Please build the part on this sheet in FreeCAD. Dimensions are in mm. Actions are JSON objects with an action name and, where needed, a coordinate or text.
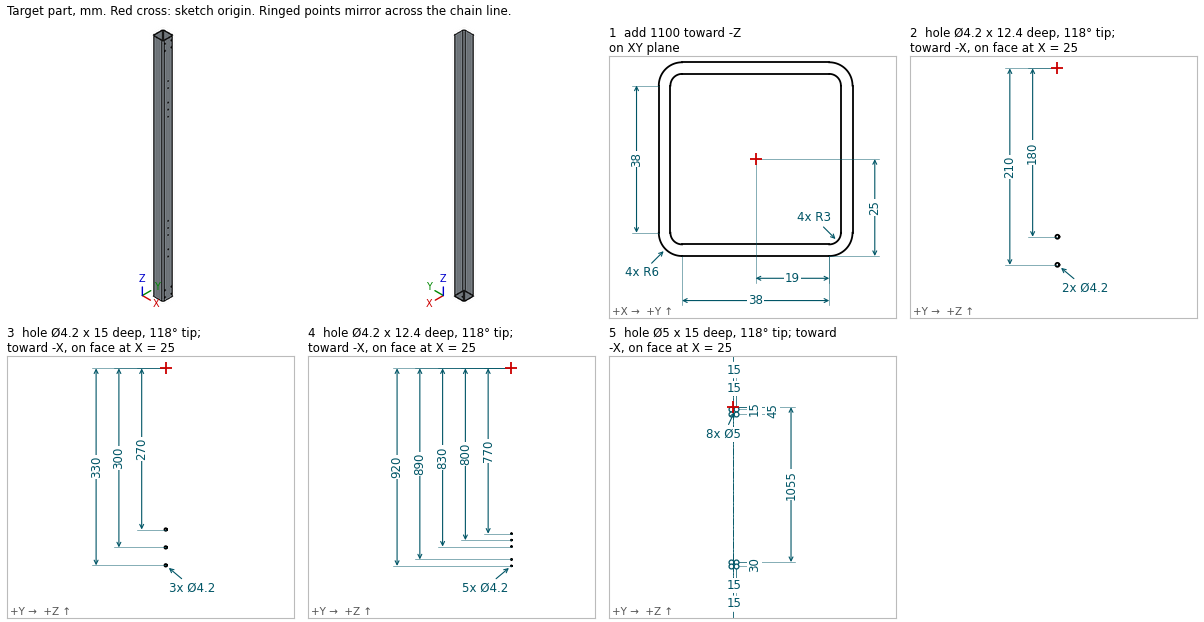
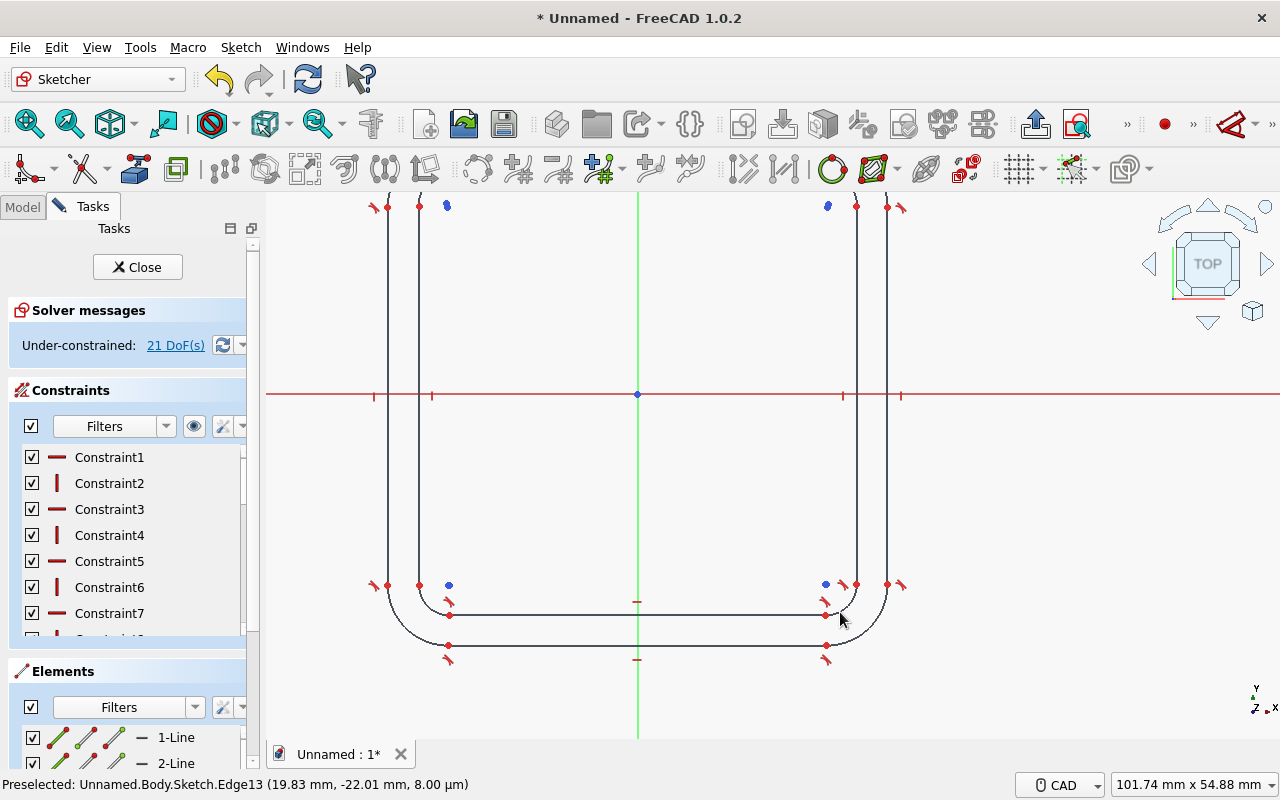
{"action": "left_click", "coordinate": [857, 471]}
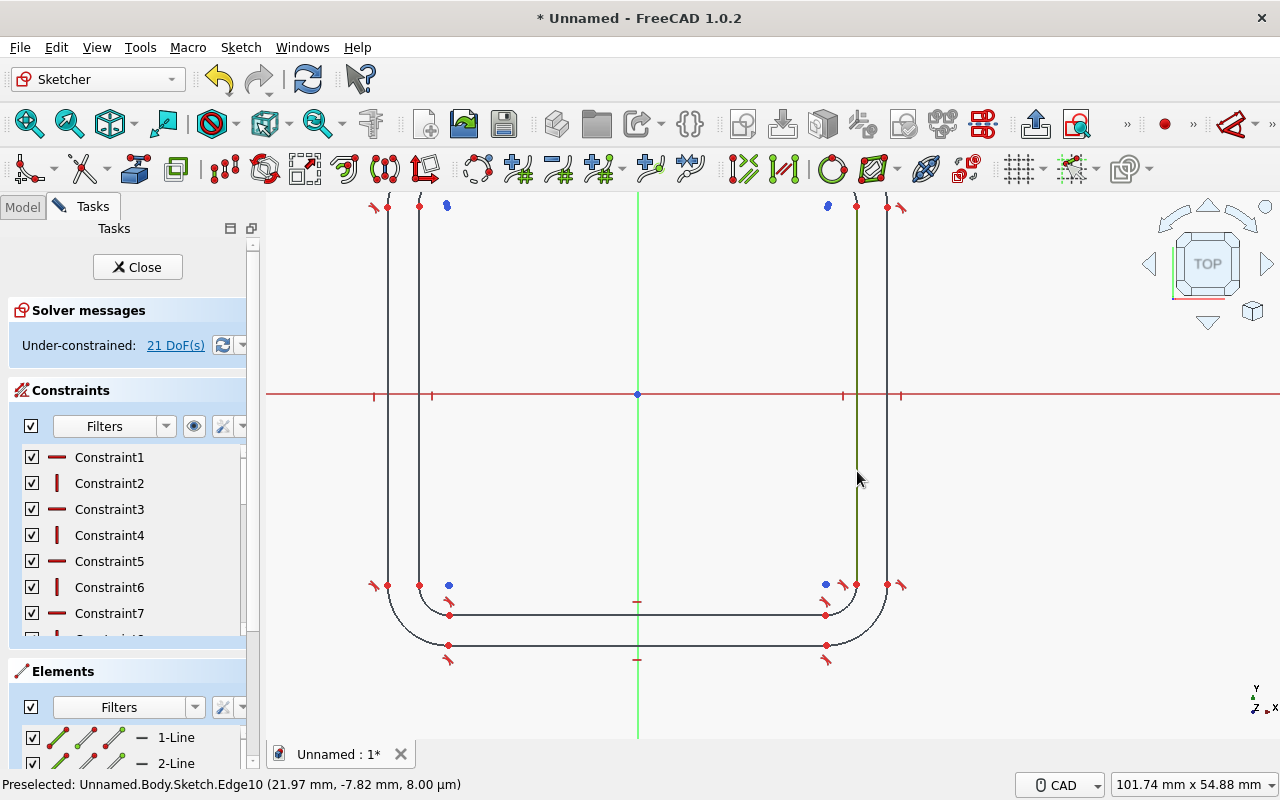
{"action": "scroll", "coordinate": [840, 611], "scroll_direction": "down", "scroll_amount": 2}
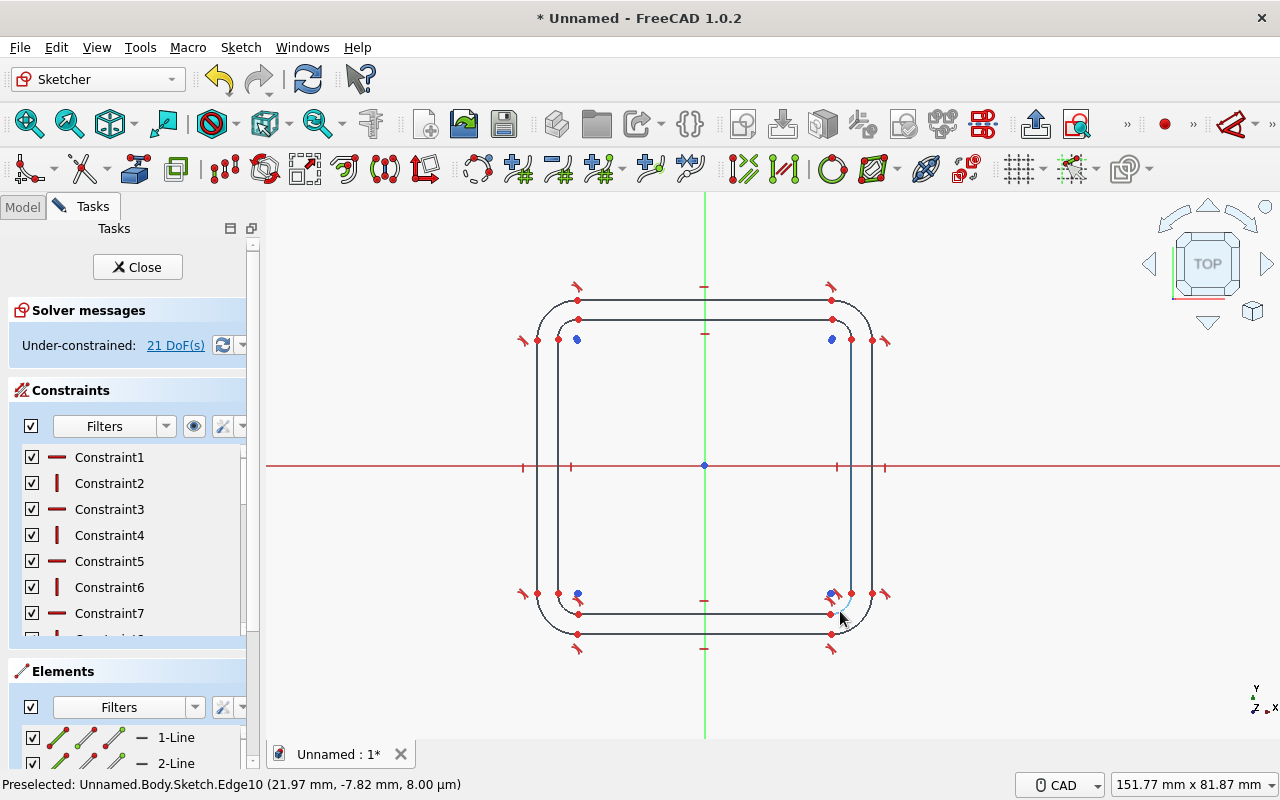
{"action": "scroll", "coordinate": [850, 331], "scroll_direction": "up", "scroll_amount": 2}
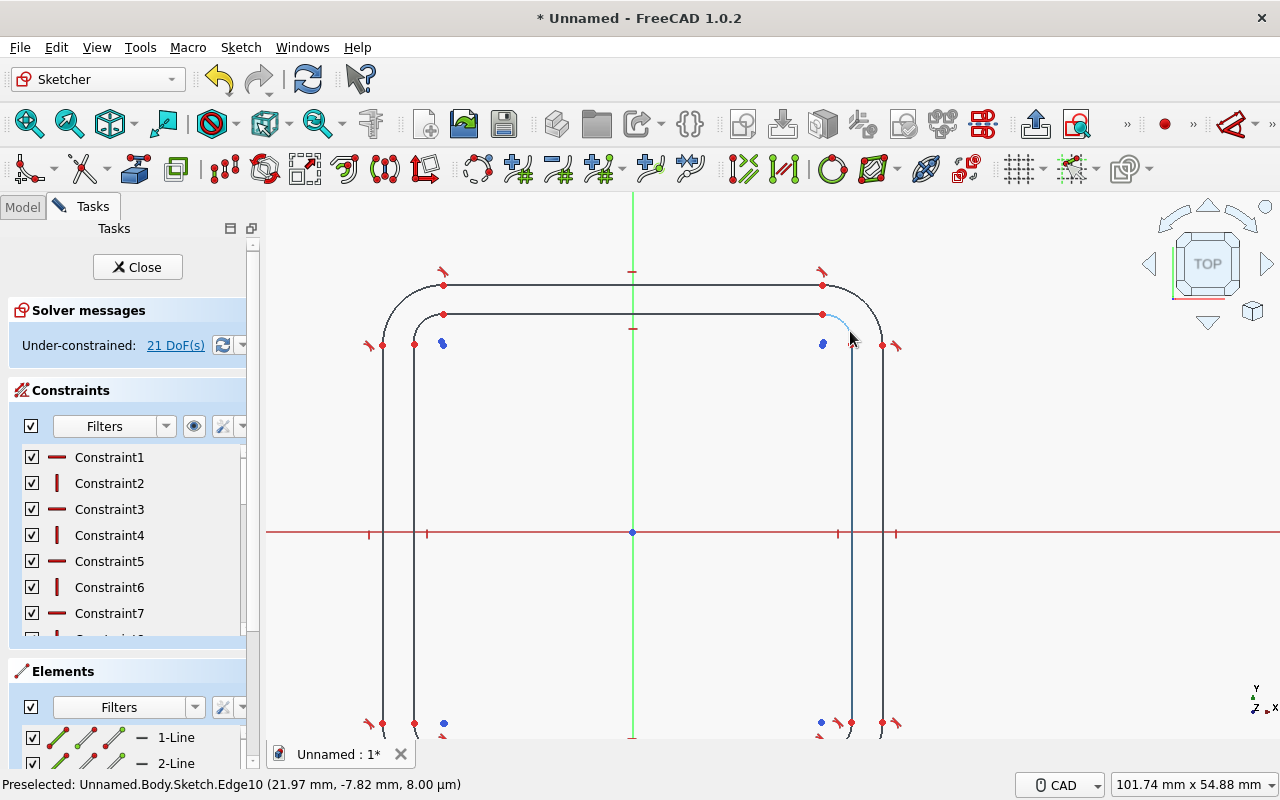
{"action": "left_click", "coordinate": [849, 331]}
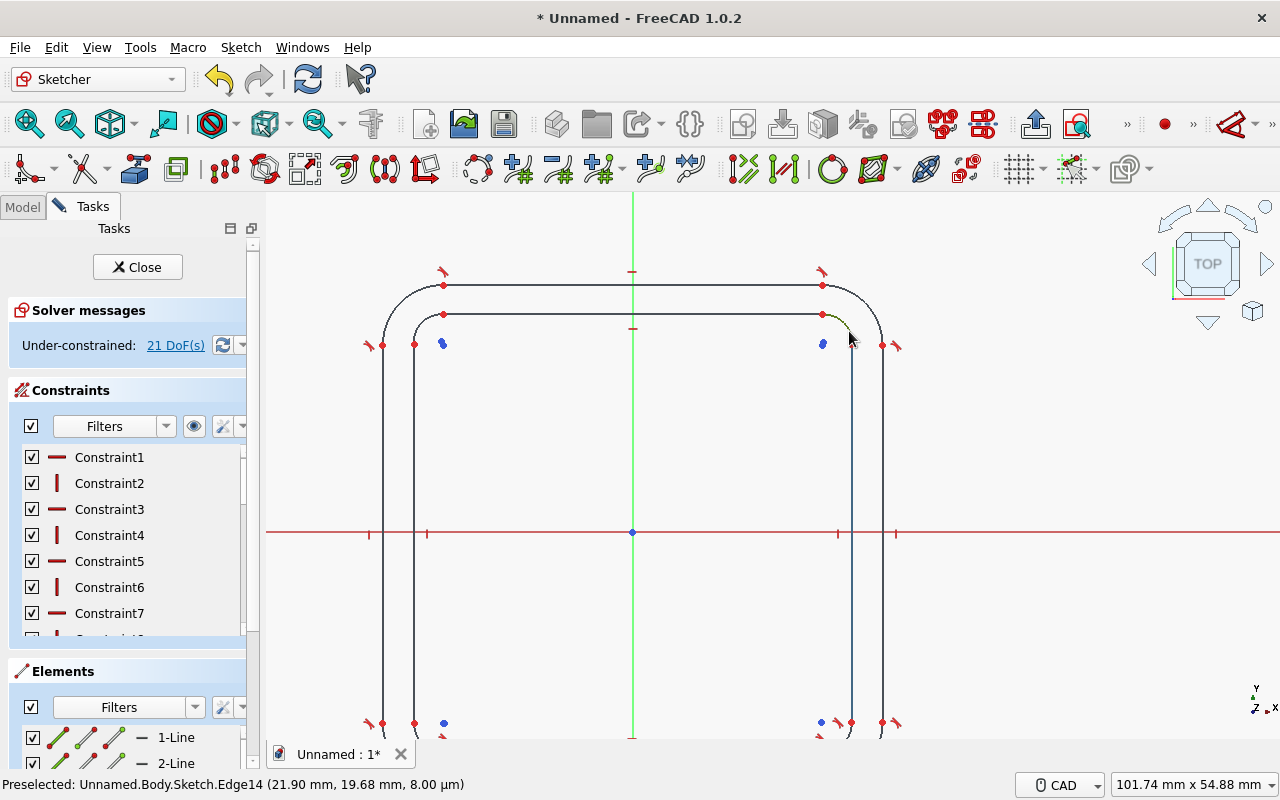
{"action": "key", "text": "t"}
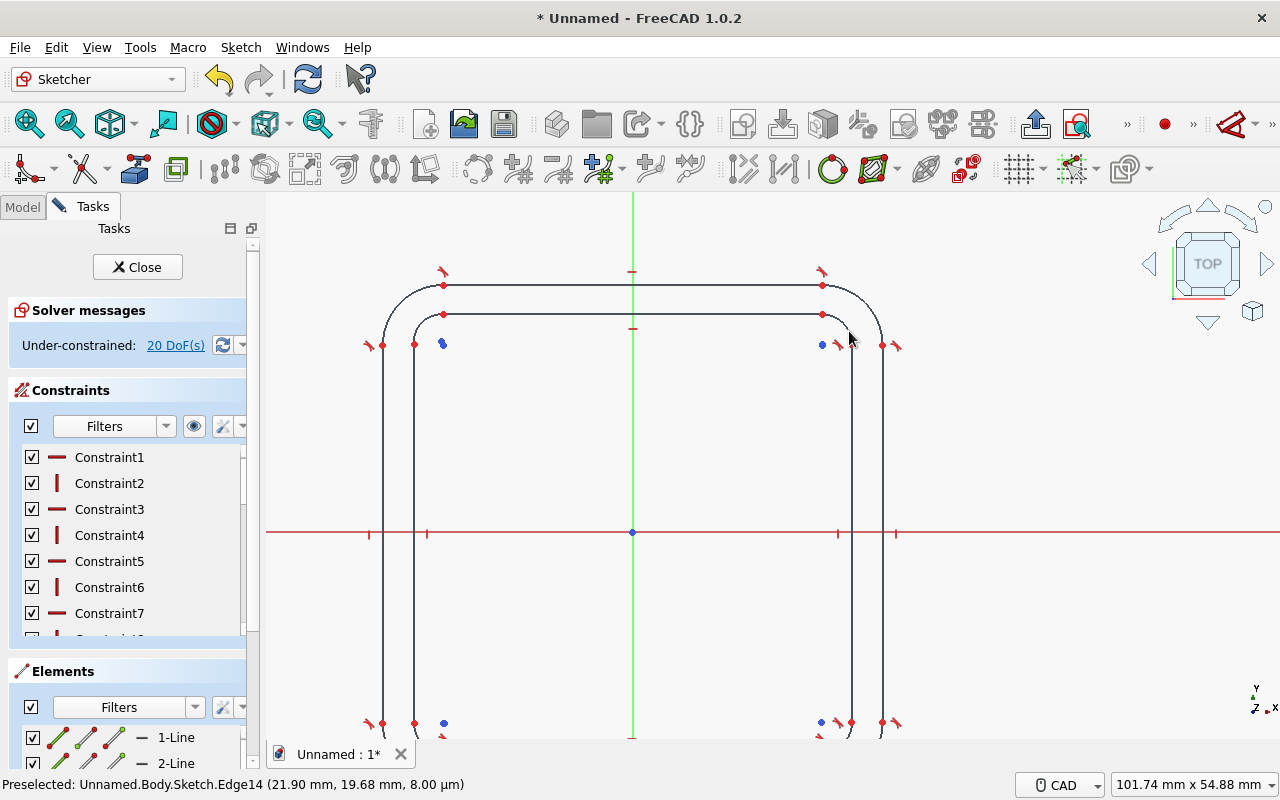
{"action": "left_click", "coordinate": [709, 314]}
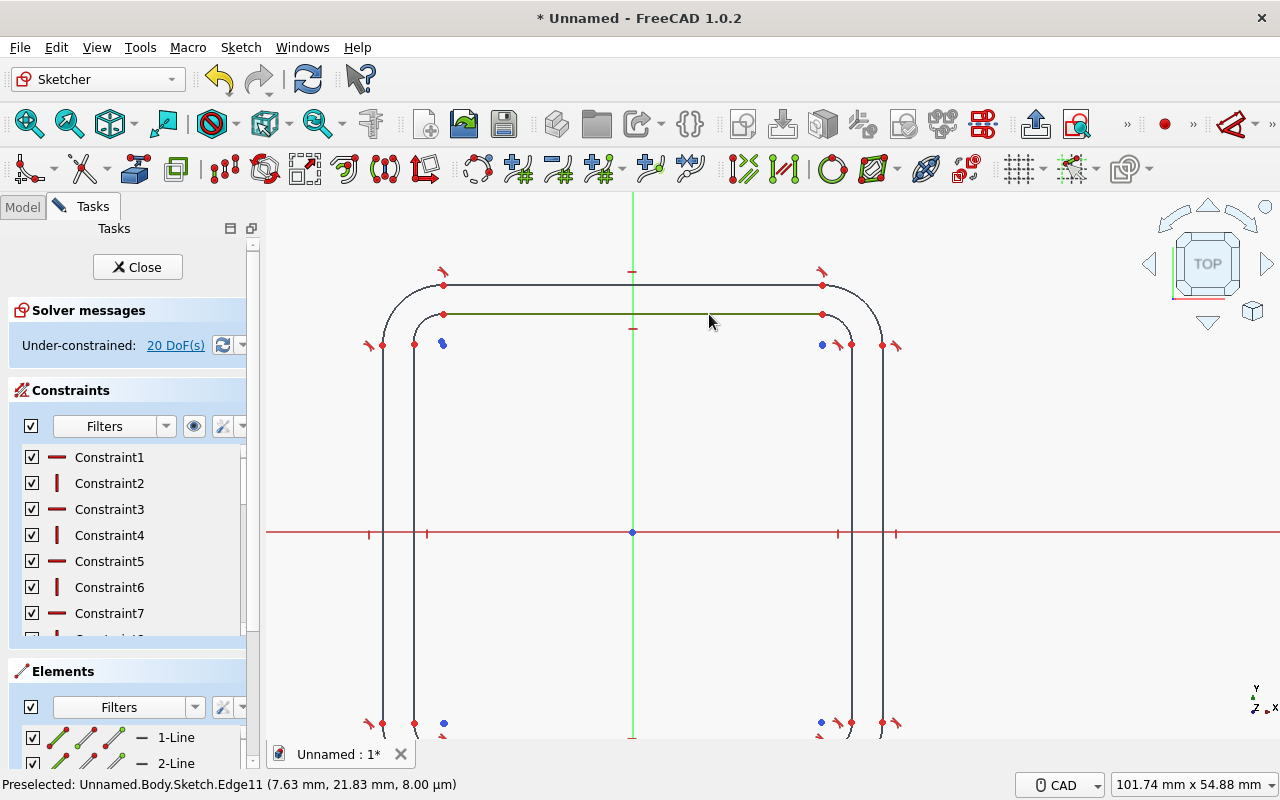
{"action": "left_click", "coordinate": [849, 331]}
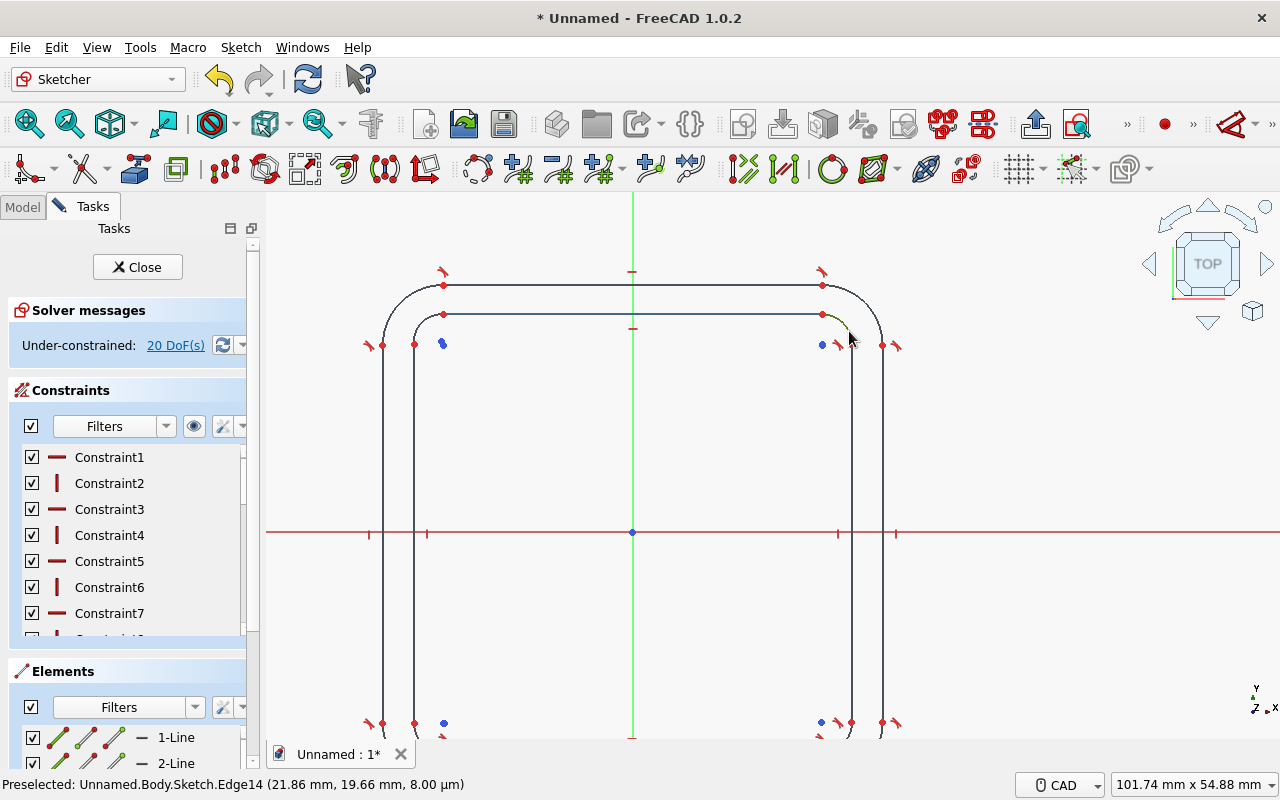
{"action": "key", "text": "t"}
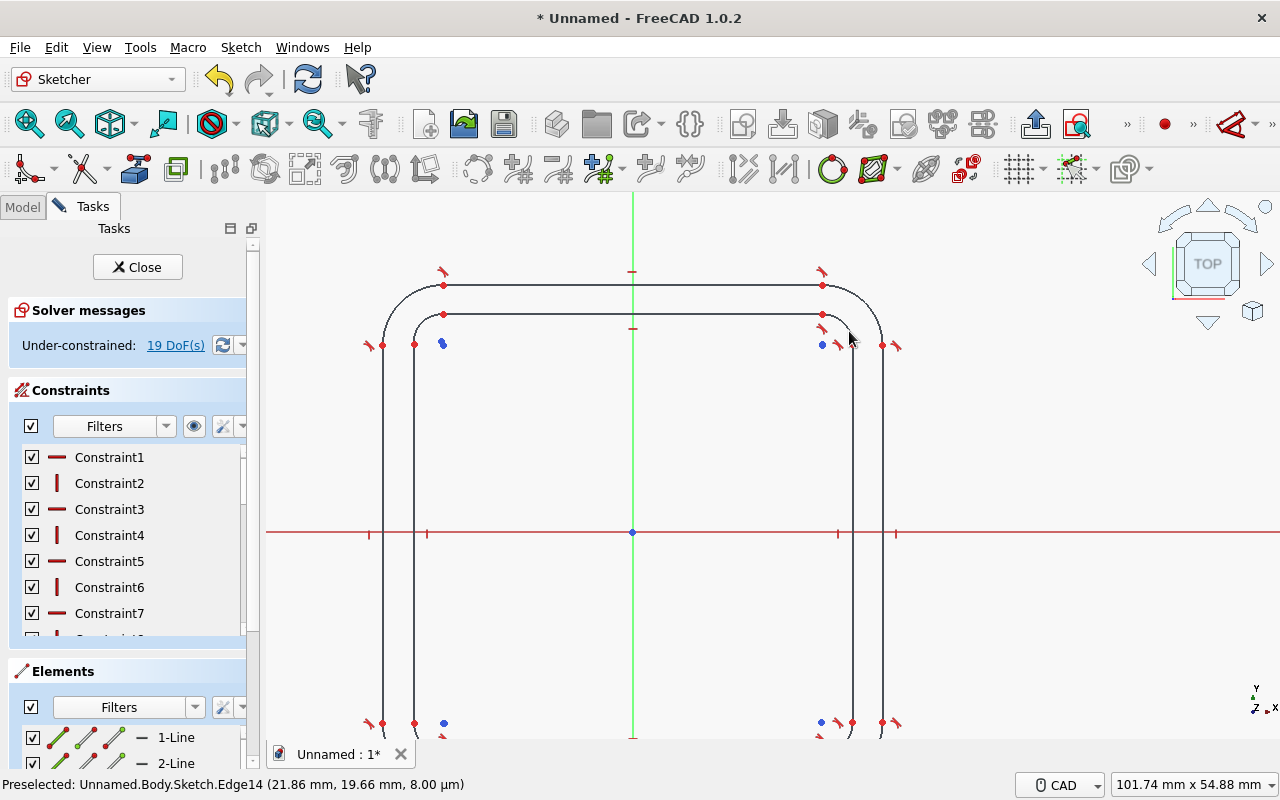
{"action": "left_click", "coordinate": [709, 314]}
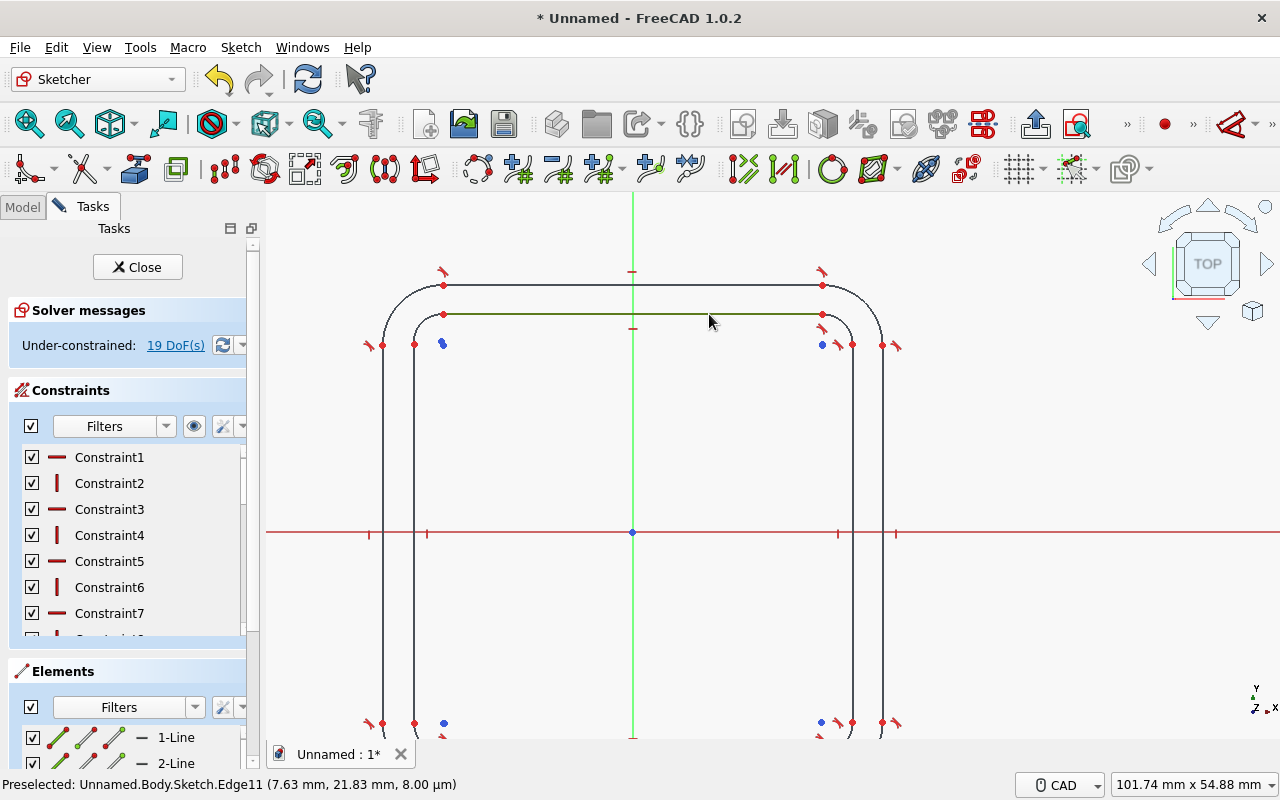
{"action": "left_click", "coordinate": [430, 317]}